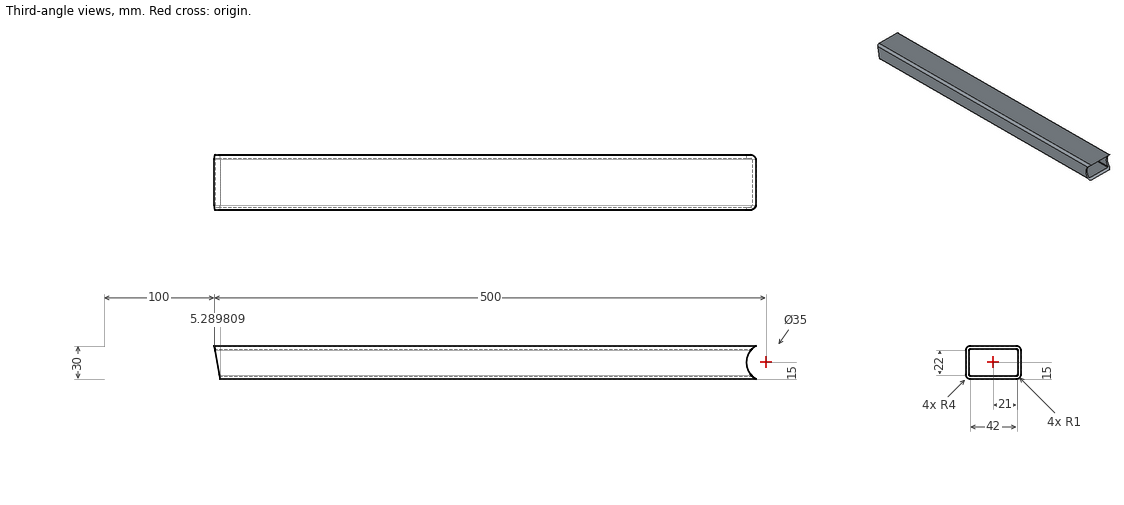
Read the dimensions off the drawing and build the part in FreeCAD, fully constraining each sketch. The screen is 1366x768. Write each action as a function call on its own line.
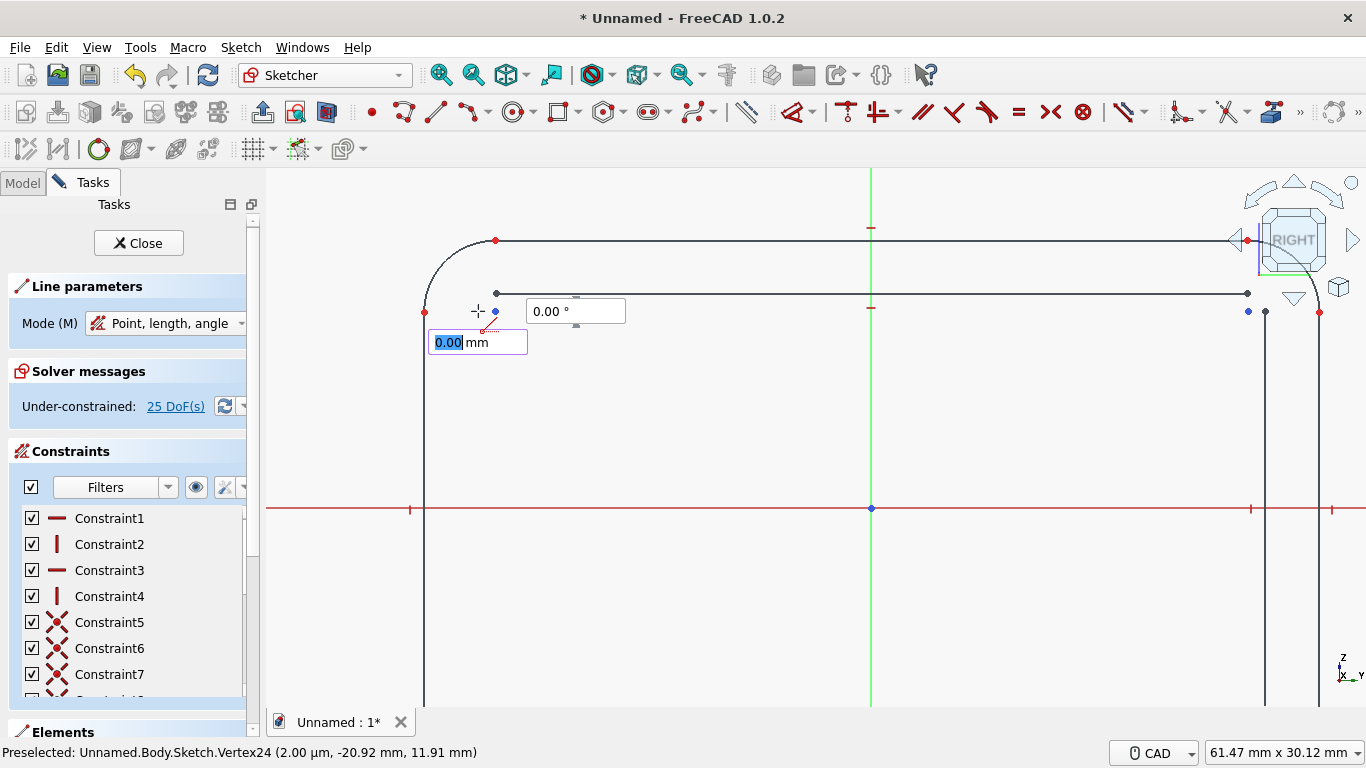
scroll(496, 294, down, 2)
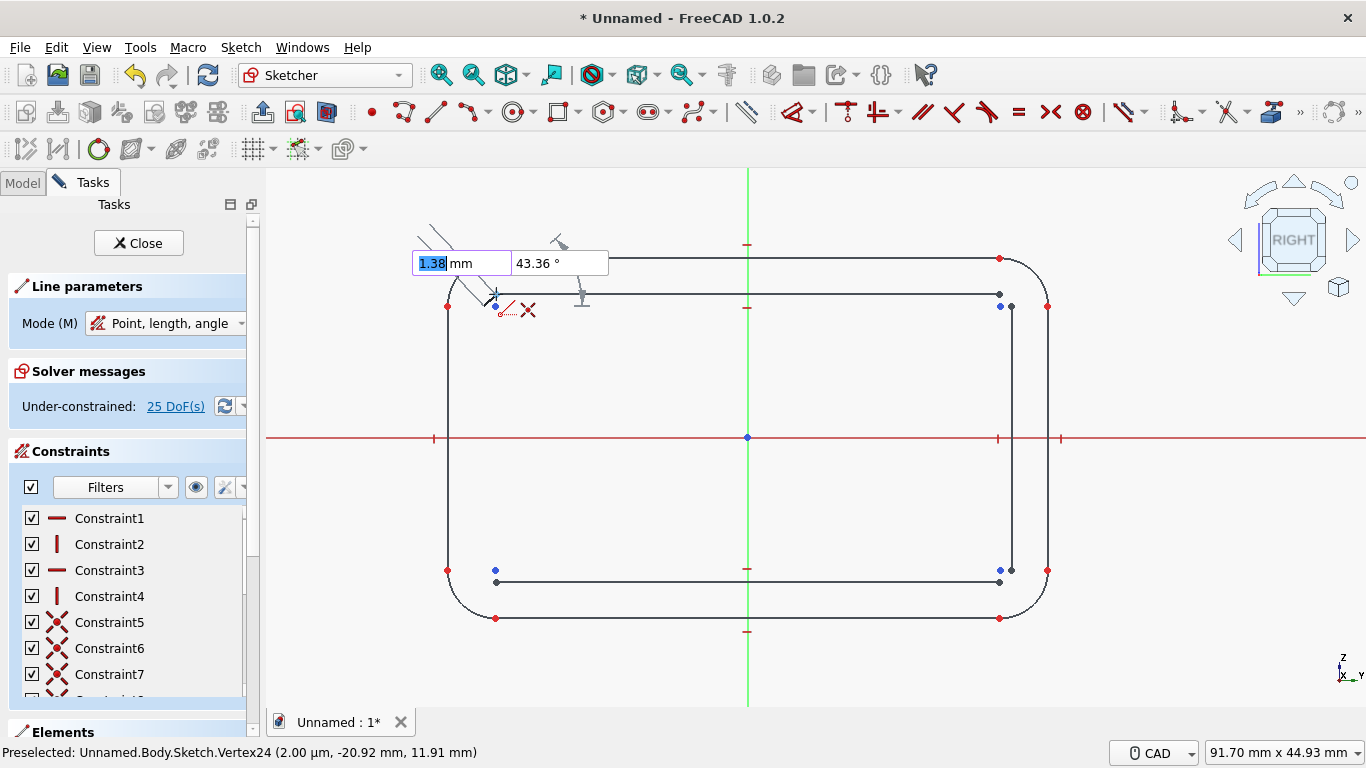
scroll(484, 570, up, 2)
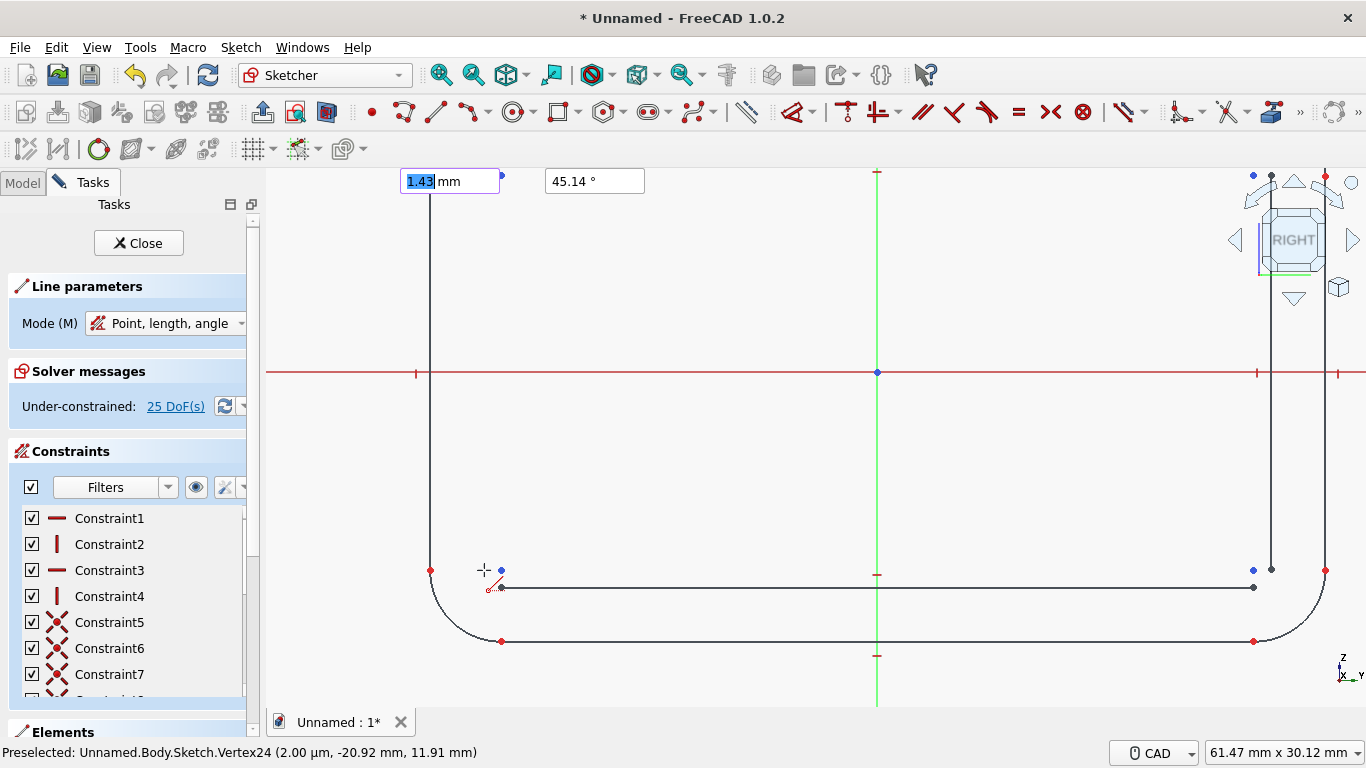
click(484, 569)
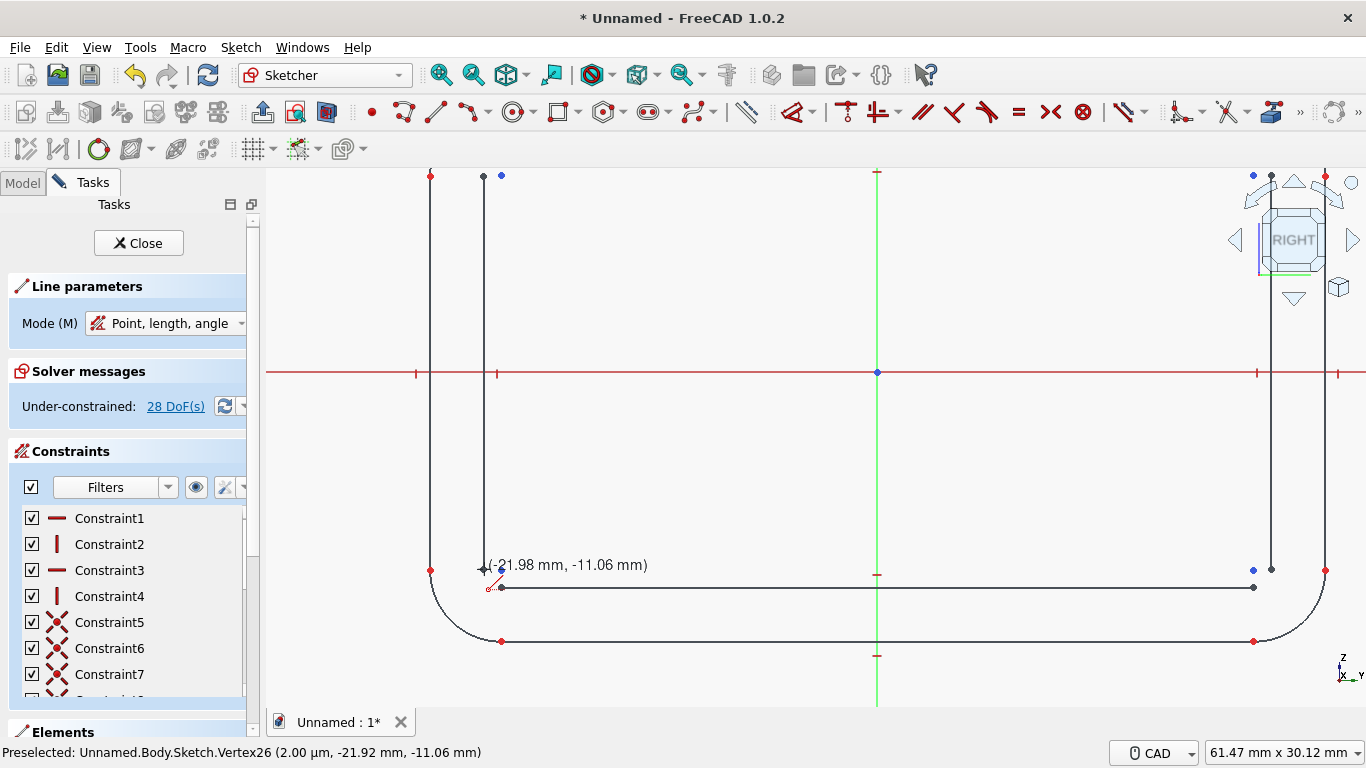
key(g)
key(3)
key(a)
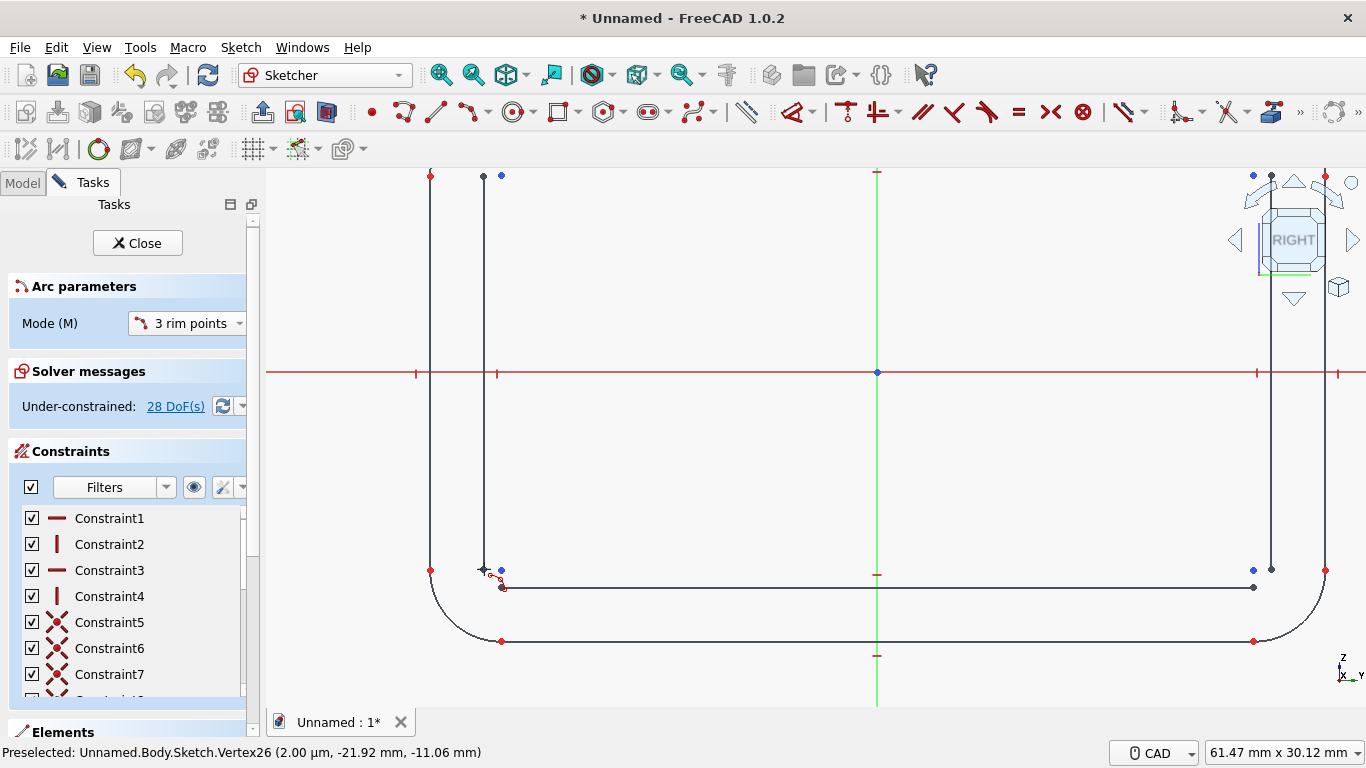
scroll(484, 570, down, 2)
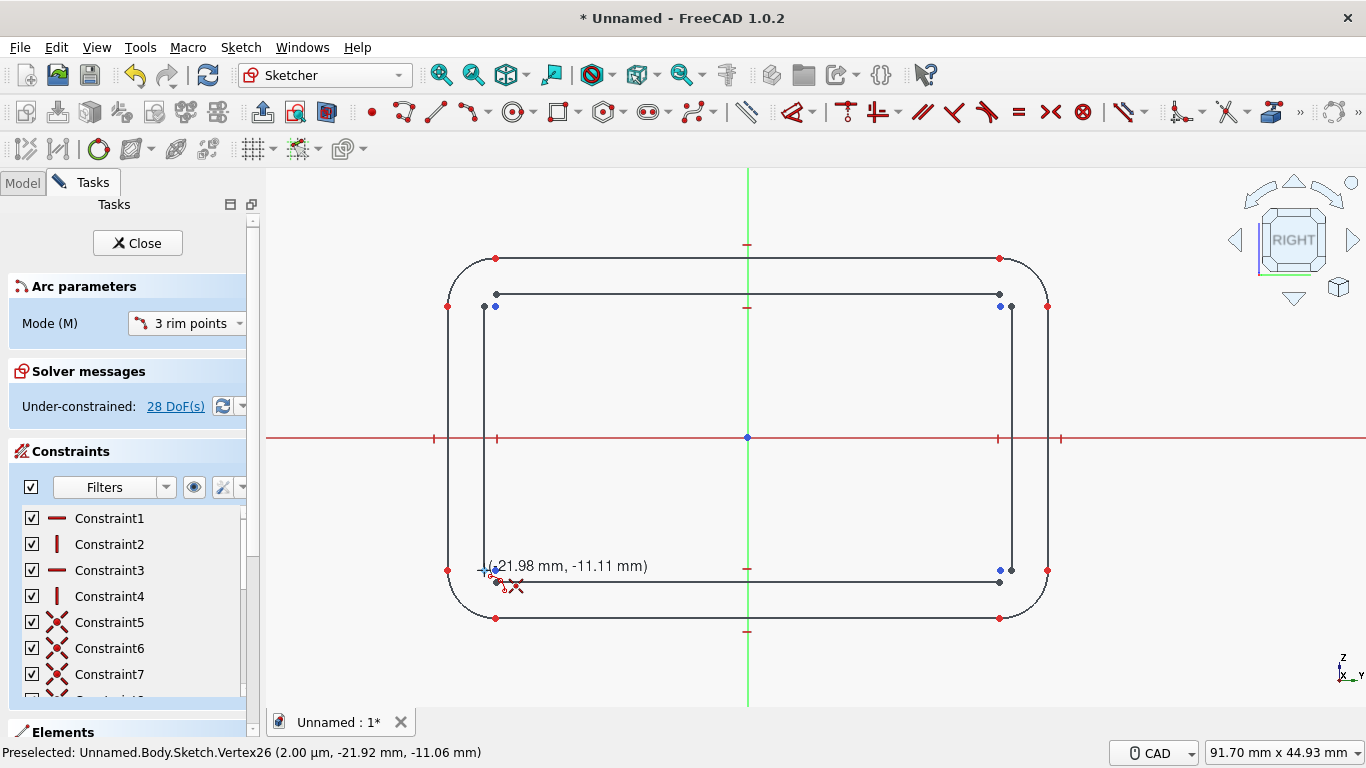
scroll(1000, 582, up, 2)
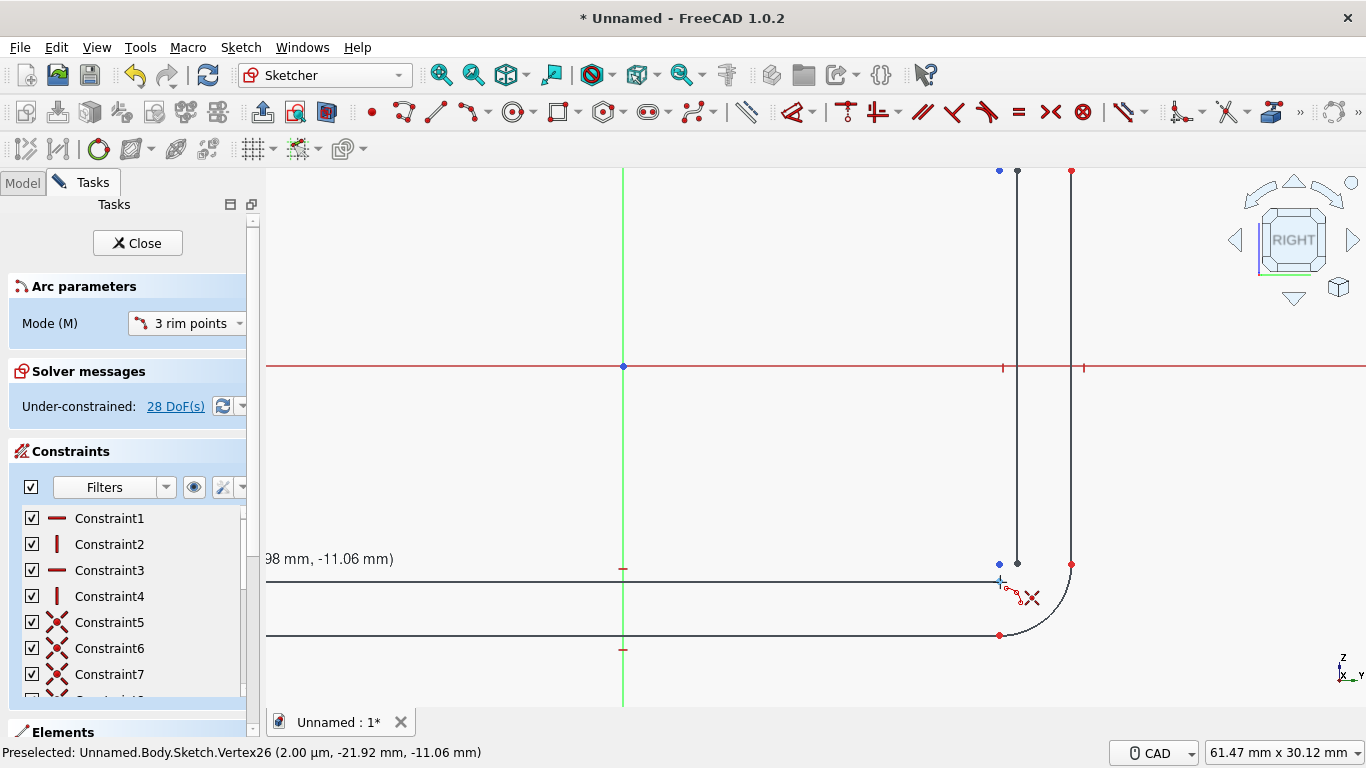
click(999, 582)
click(1017, 564)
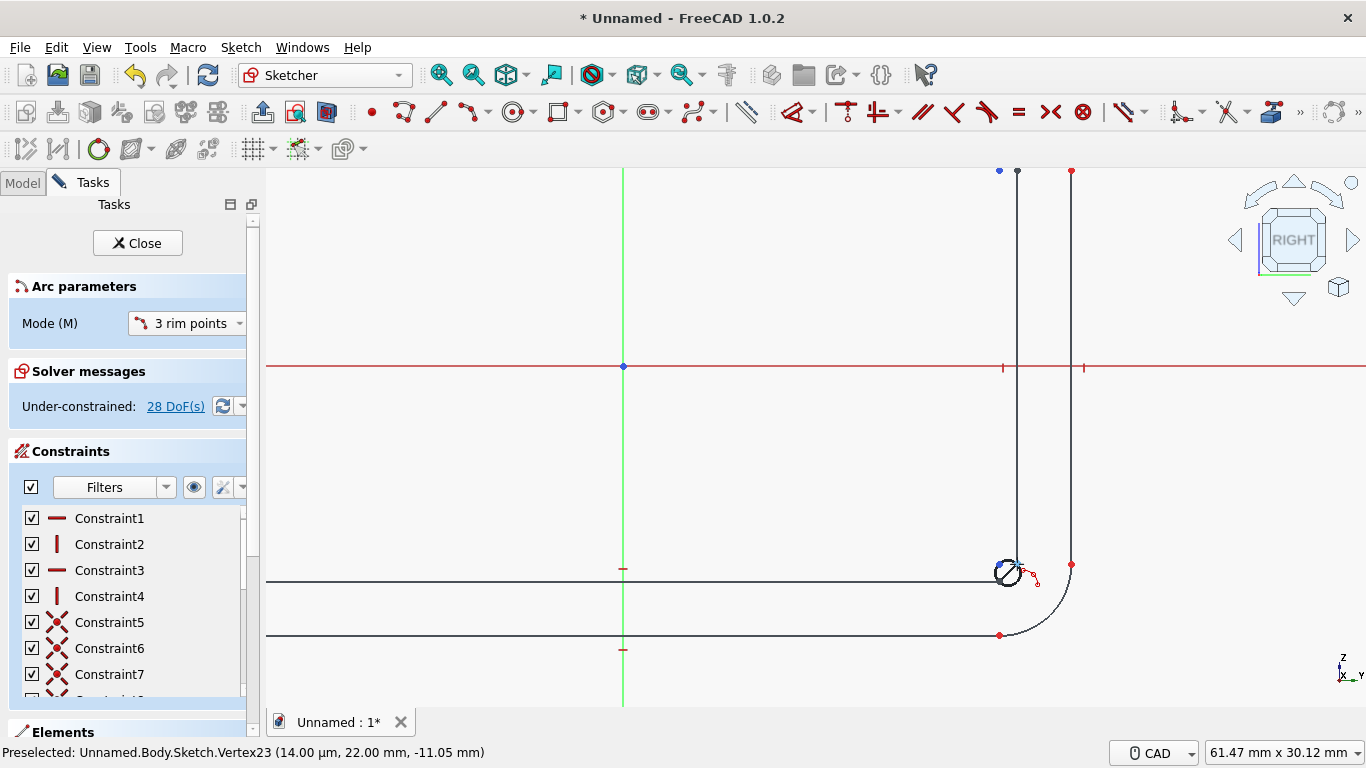
scroll(1012, 576, up, 6)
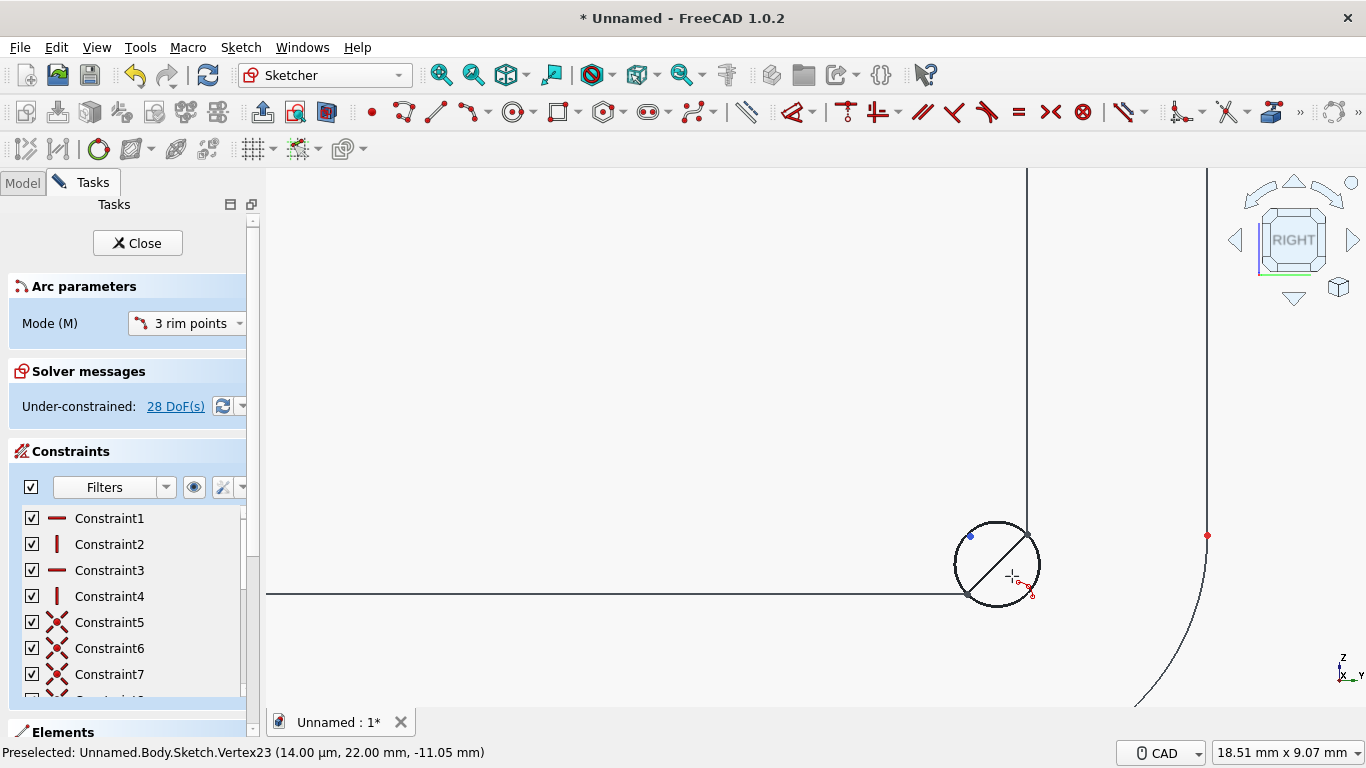
click(1009, 573)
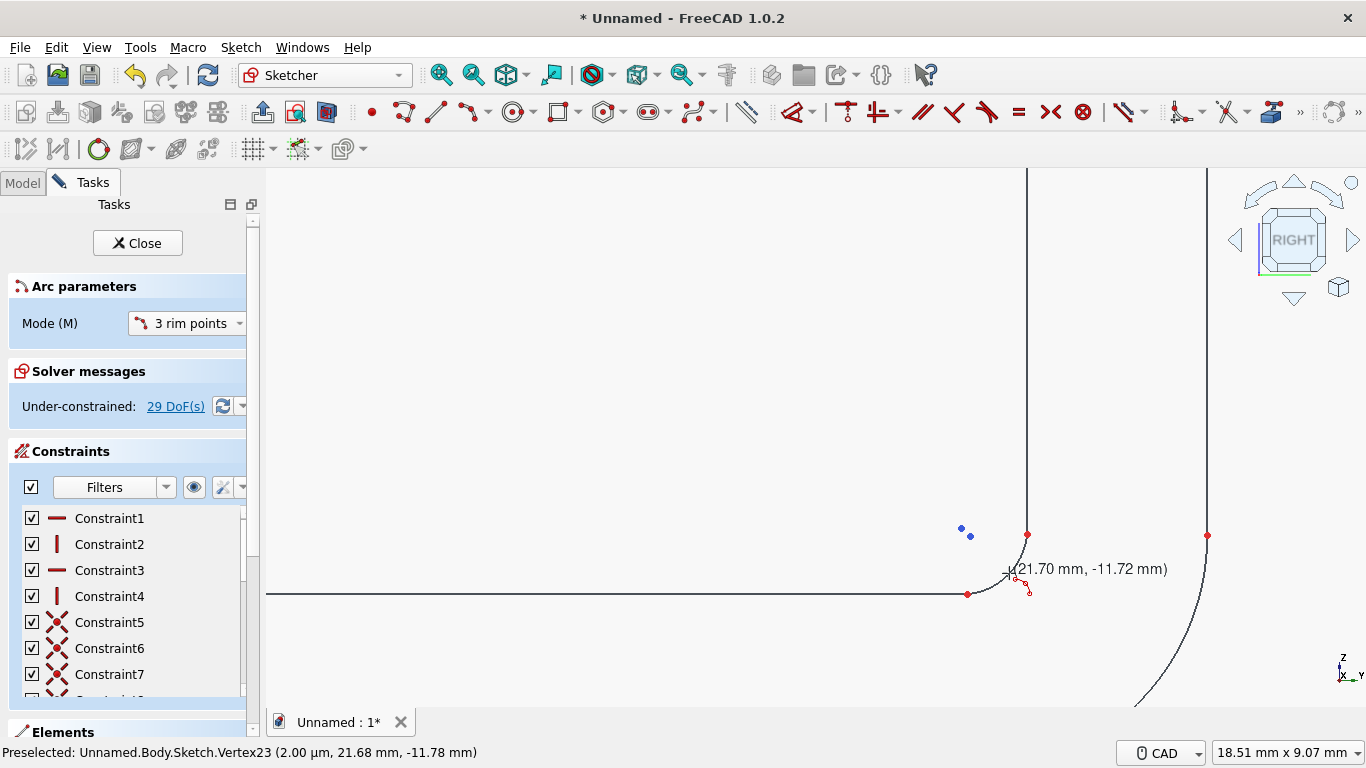
scroll(1007, 579, down, 8)